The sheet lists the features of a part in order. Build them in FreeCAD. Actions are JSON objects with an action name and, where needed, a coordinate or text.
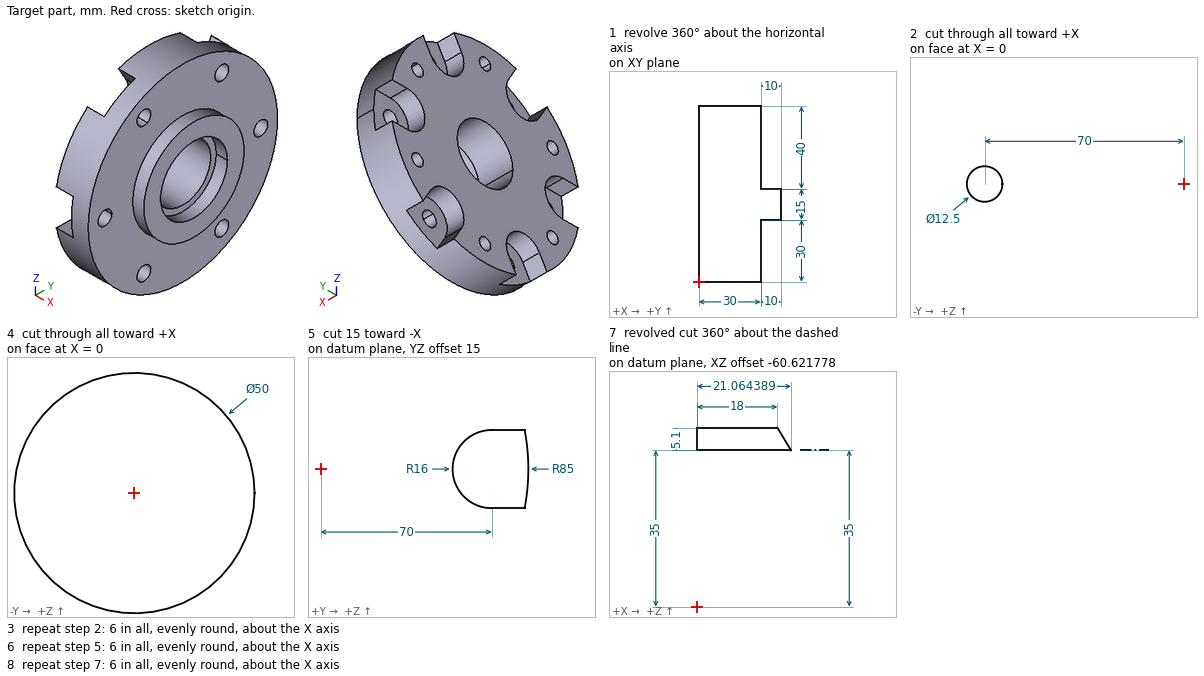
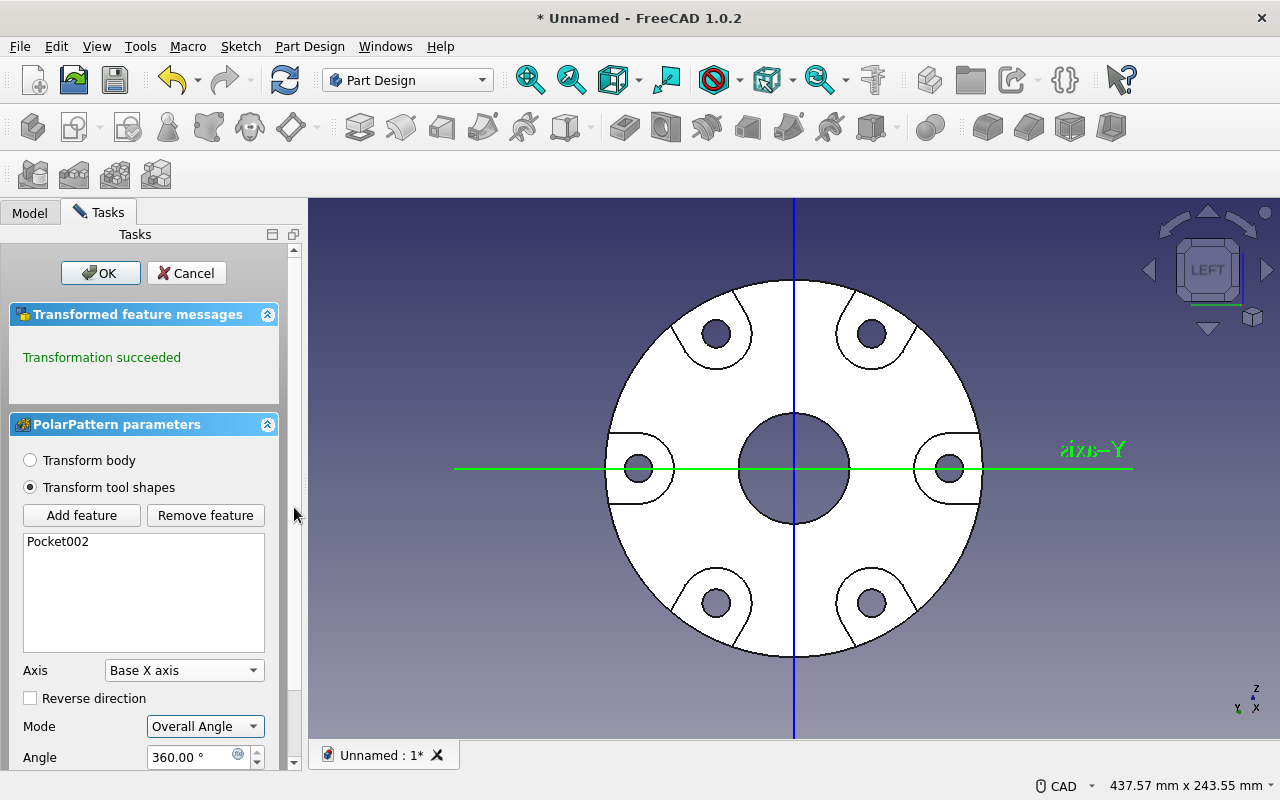
{"action": "left_click", "coordinate": [101, 273]}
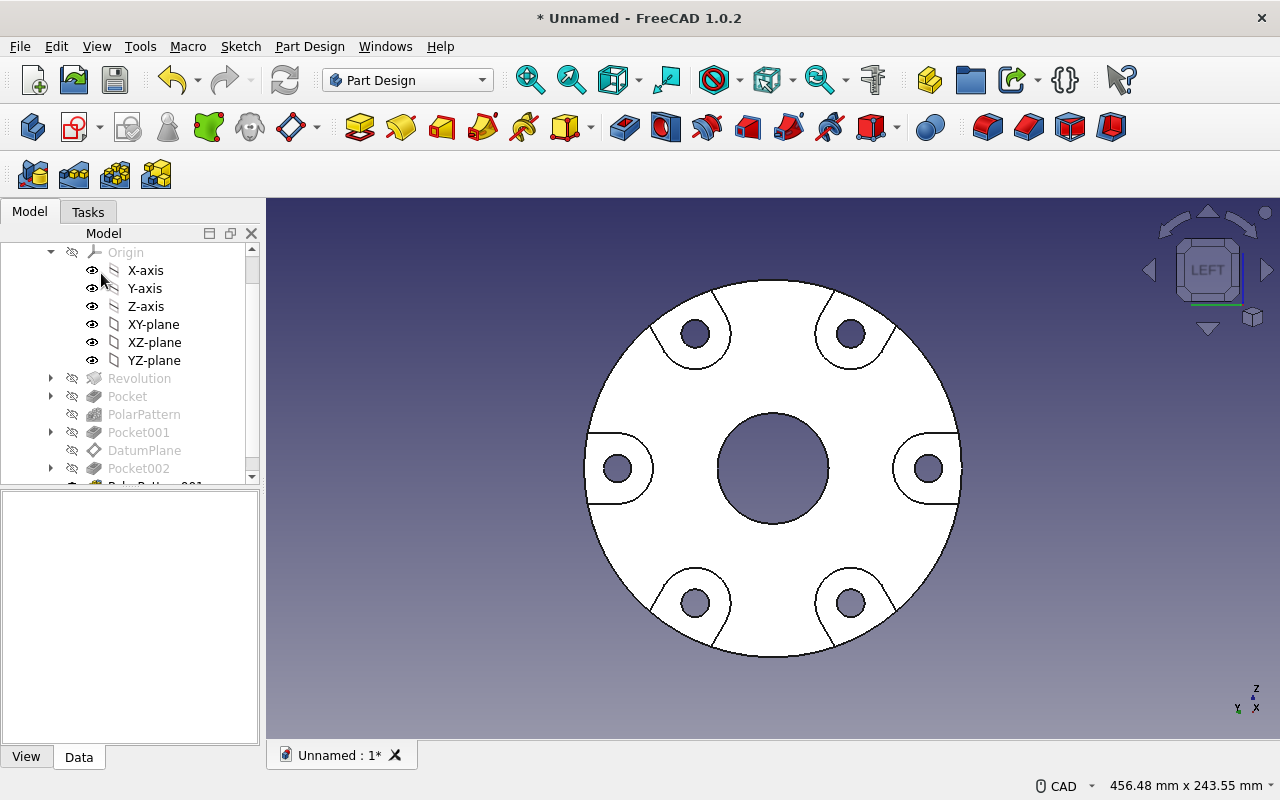
{"action": "left_click", "coordinate": [137, 342]}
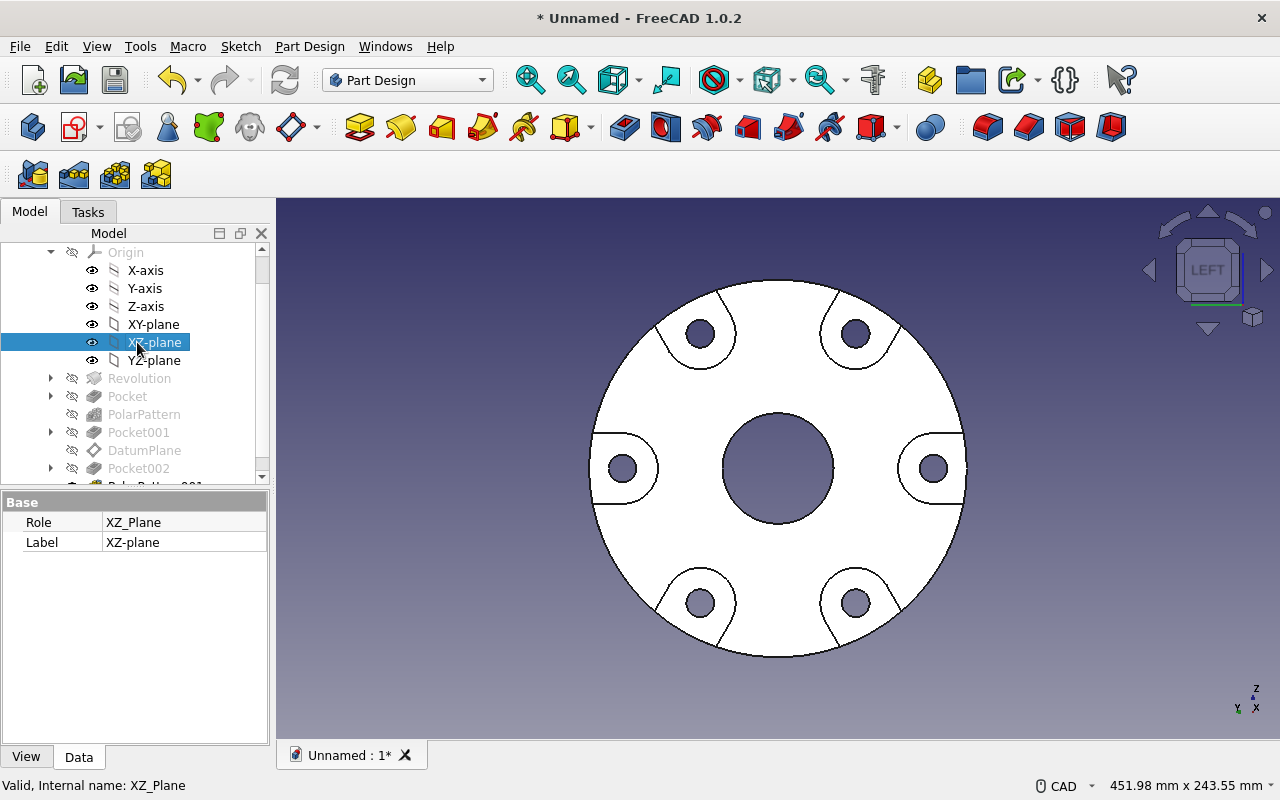
{"action": "left_click", "coordinate": [290, 128]}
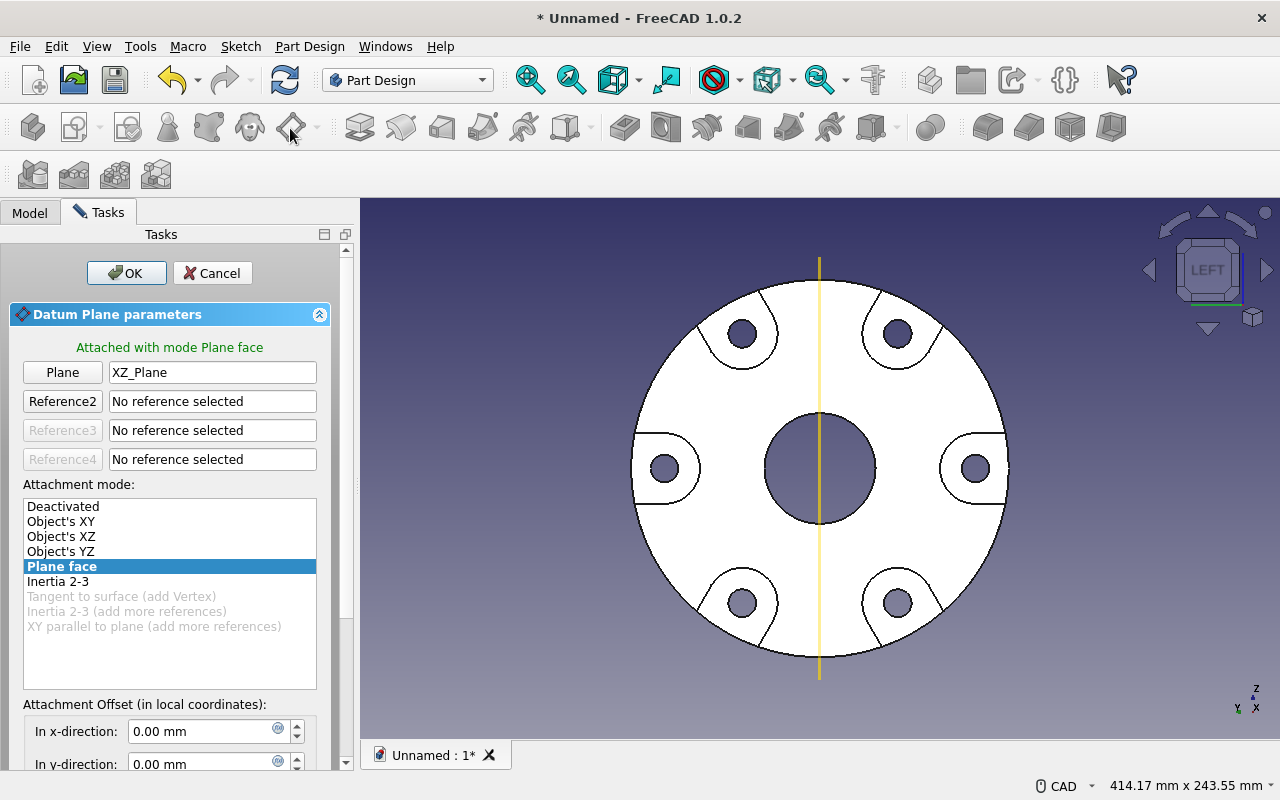
{"action": "scroll", "coordinate": [346, 507], "scroll_direction": "down", "scroll_amount": 2}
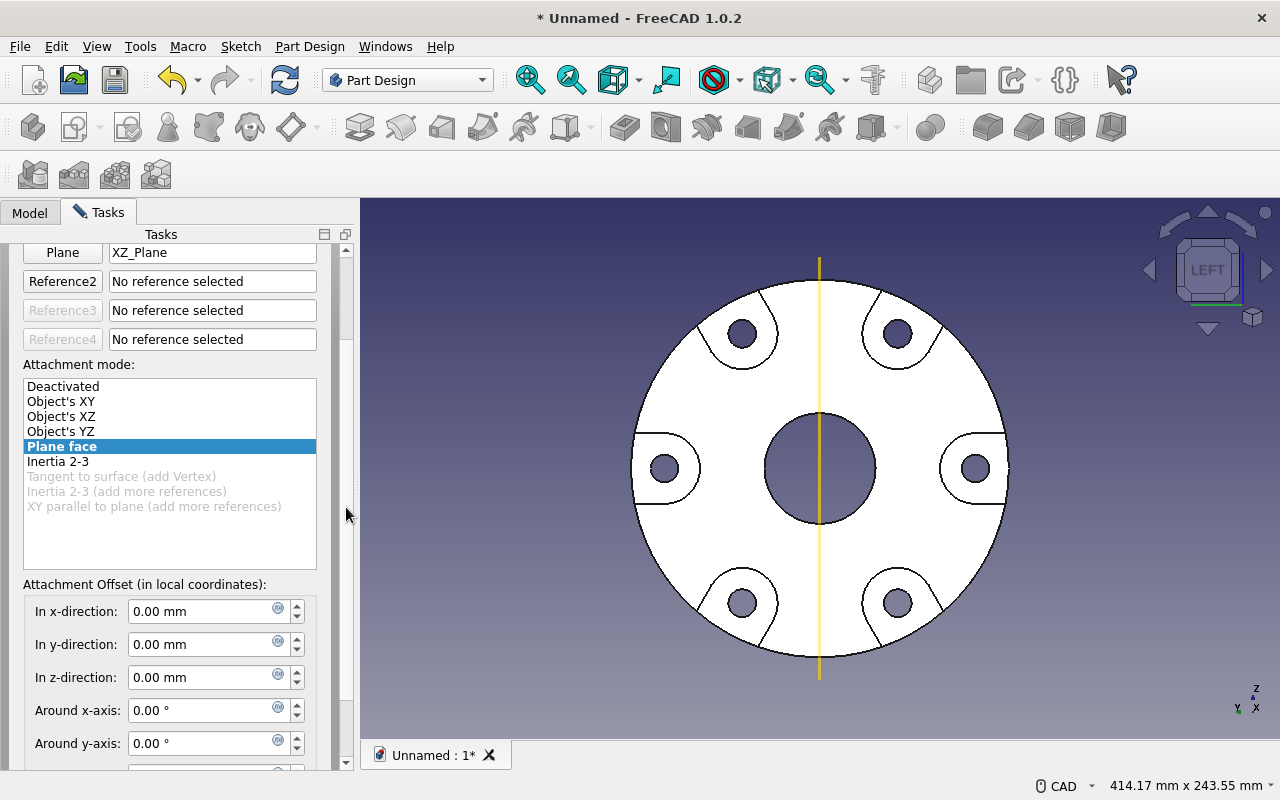
{"action": "triple_click", "coordinate": [210, 678]}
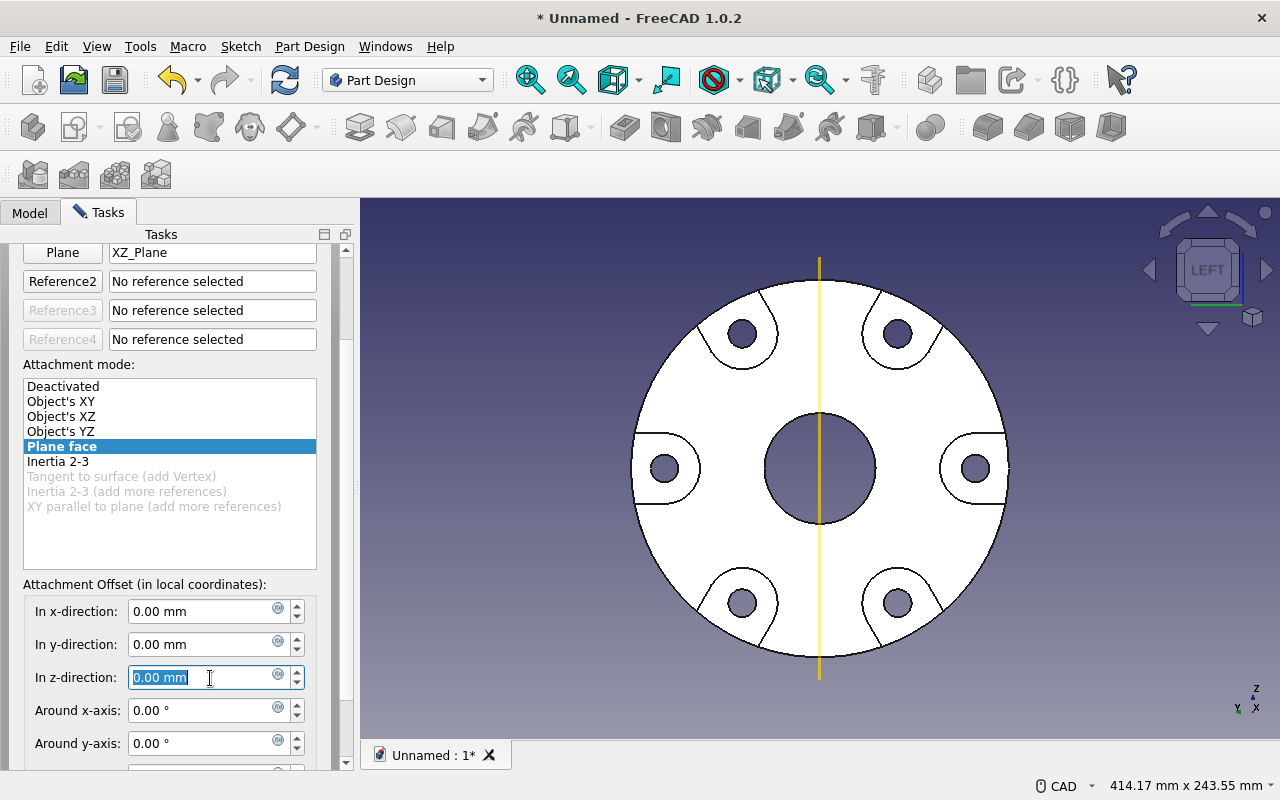
{"action": "type", "text": "-60.621778"}
{"action": "key", "text": "Tab"}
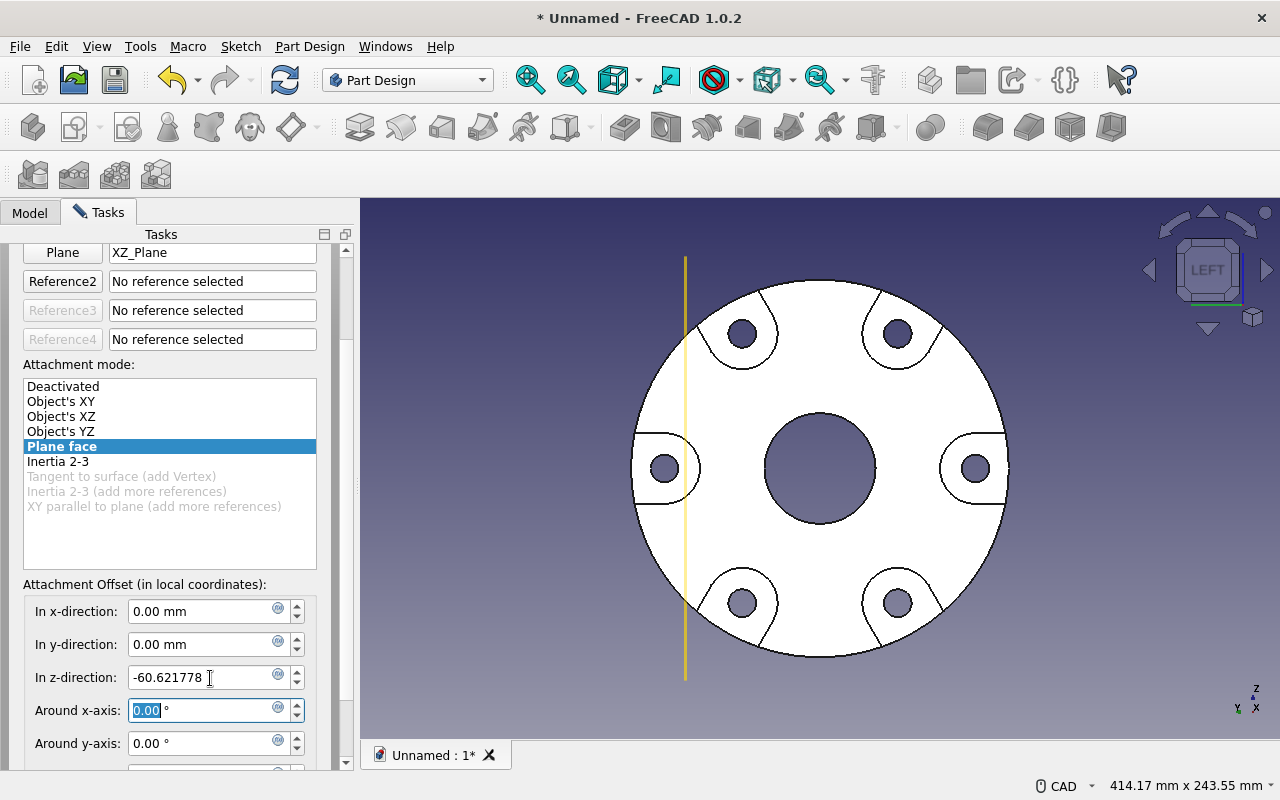
{"action": "scroll", "coordinate": [346, 507], "scroll_direction": "up", "scroll_amount": 3}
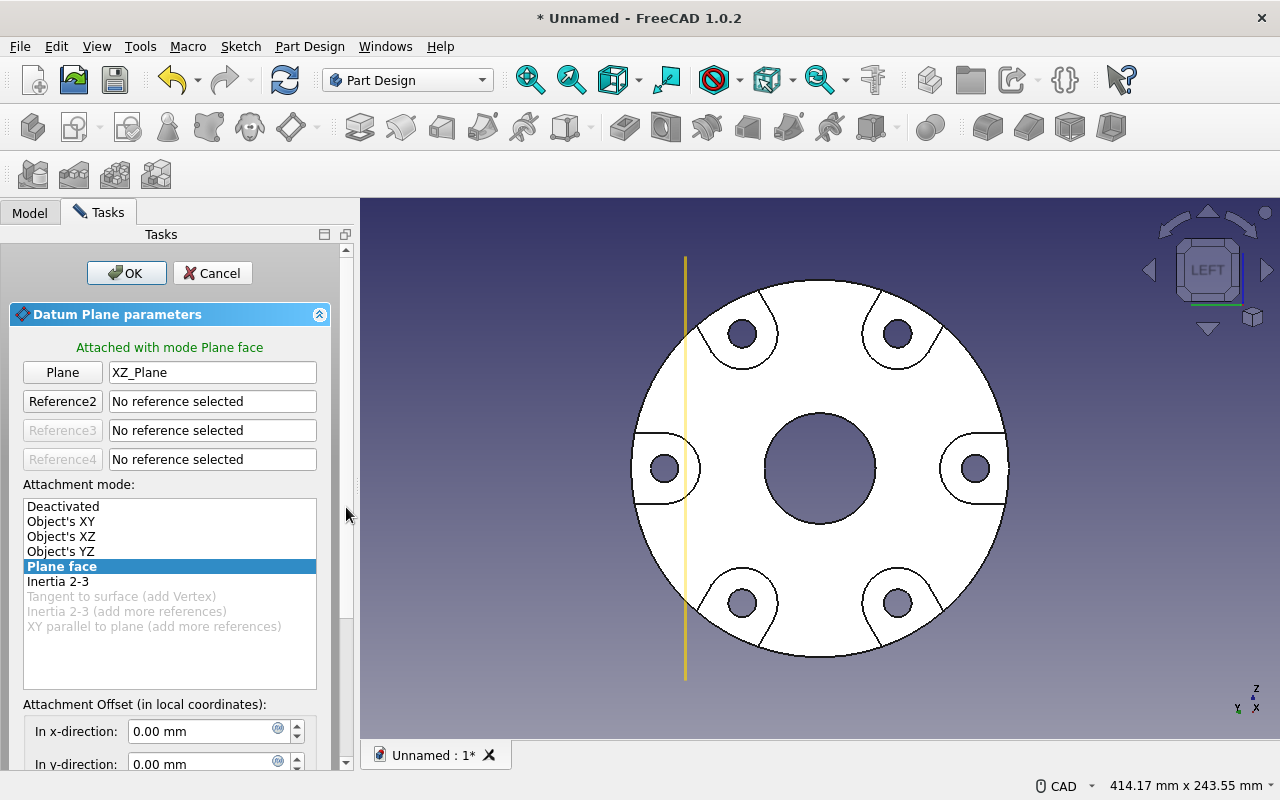
{"action": "left_click", "coordinate": [127, 273]}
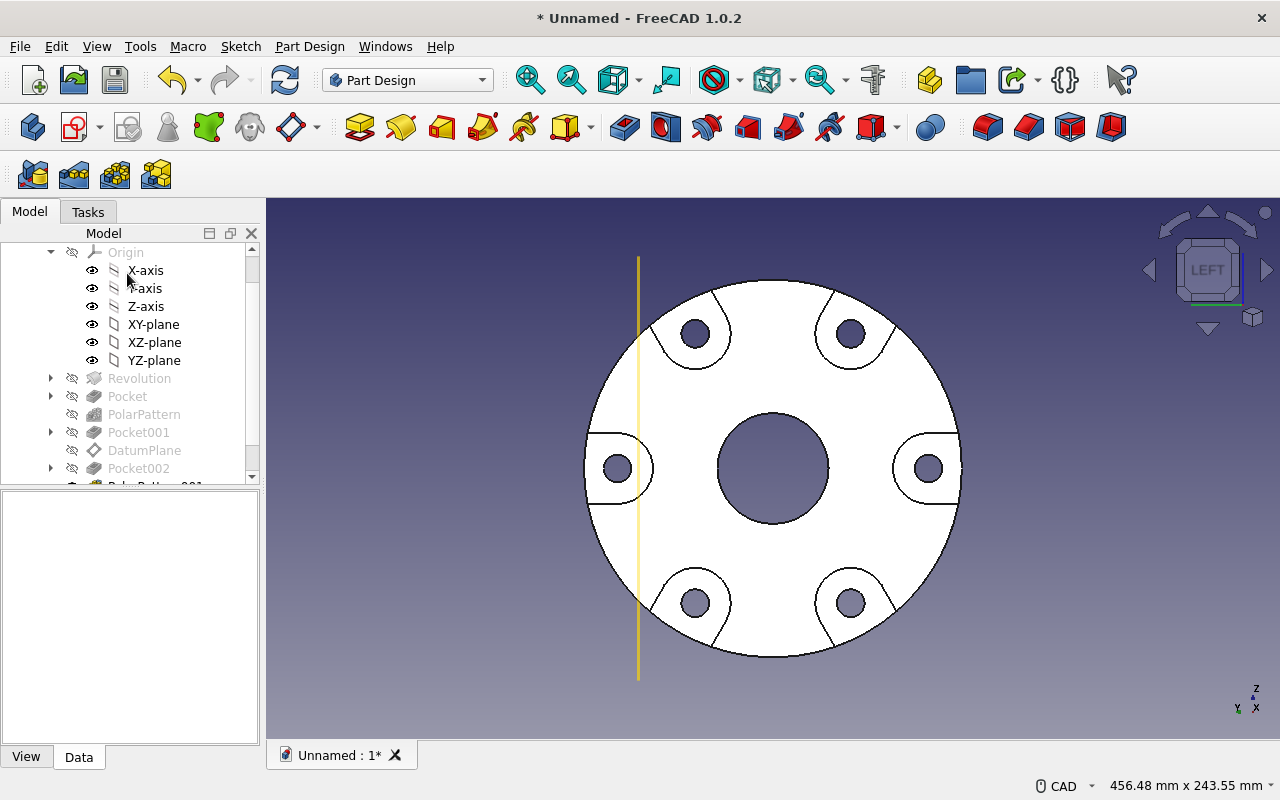
{"action": "scroll", "coordinate": [141, 356], "scroll_direction": "down", "scroll_amount": 3}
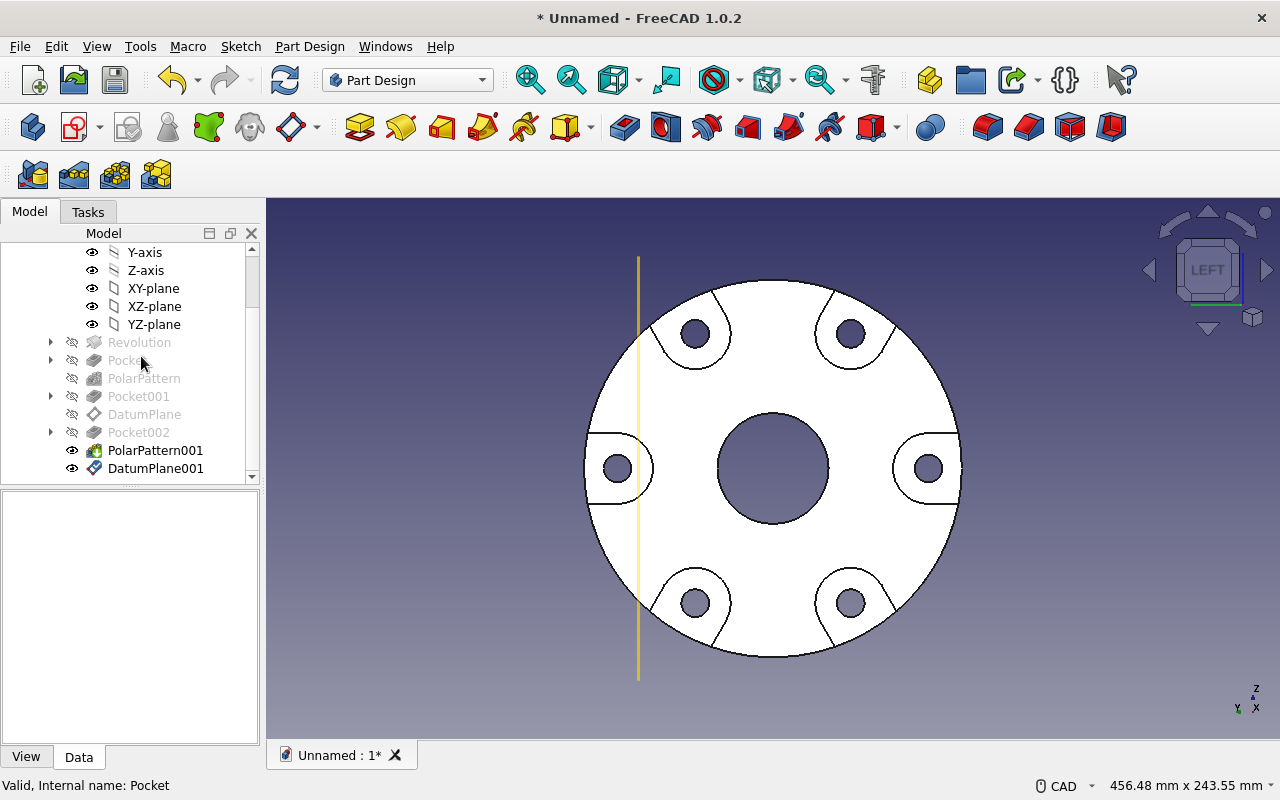
{"action": "left_click", "coordinate": [117, 468]}